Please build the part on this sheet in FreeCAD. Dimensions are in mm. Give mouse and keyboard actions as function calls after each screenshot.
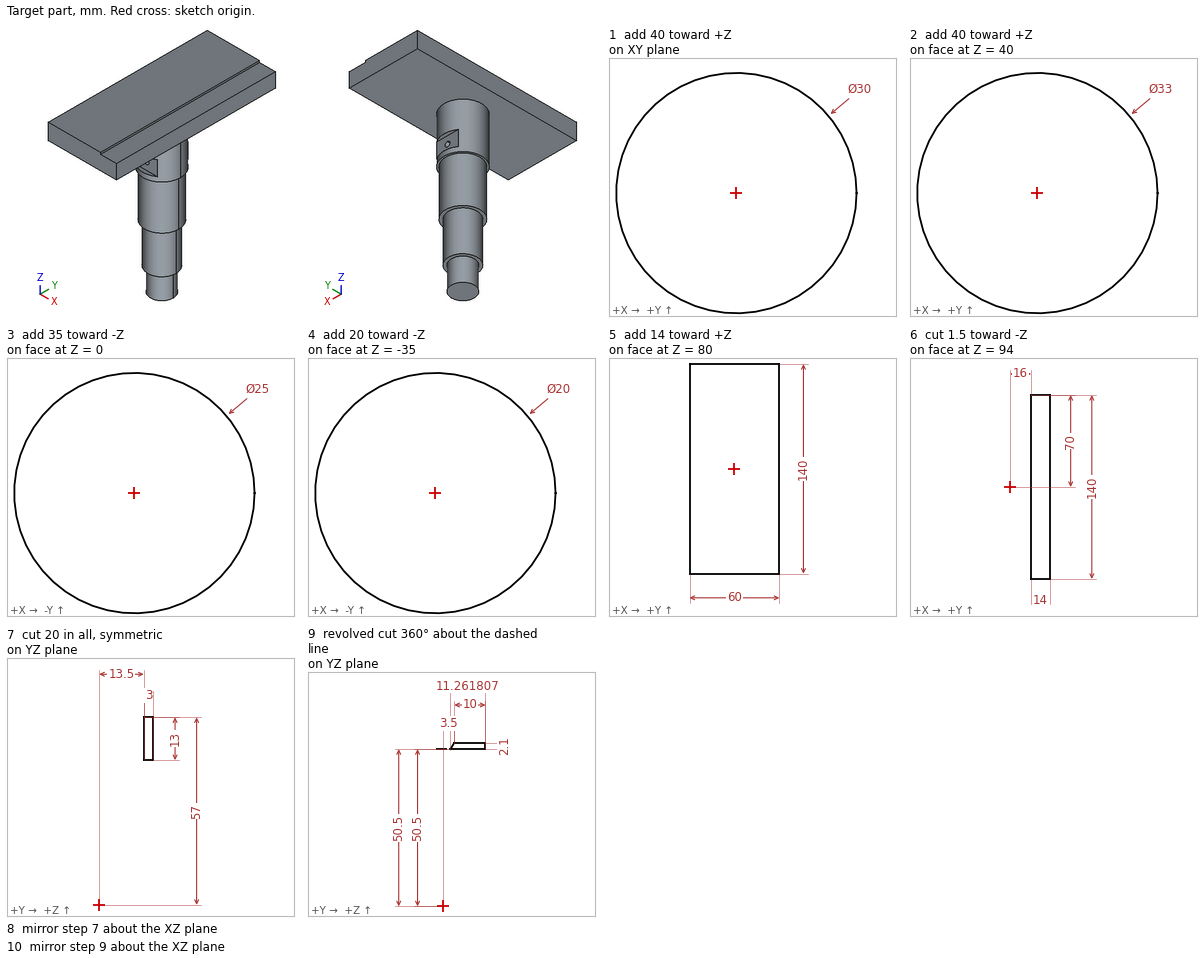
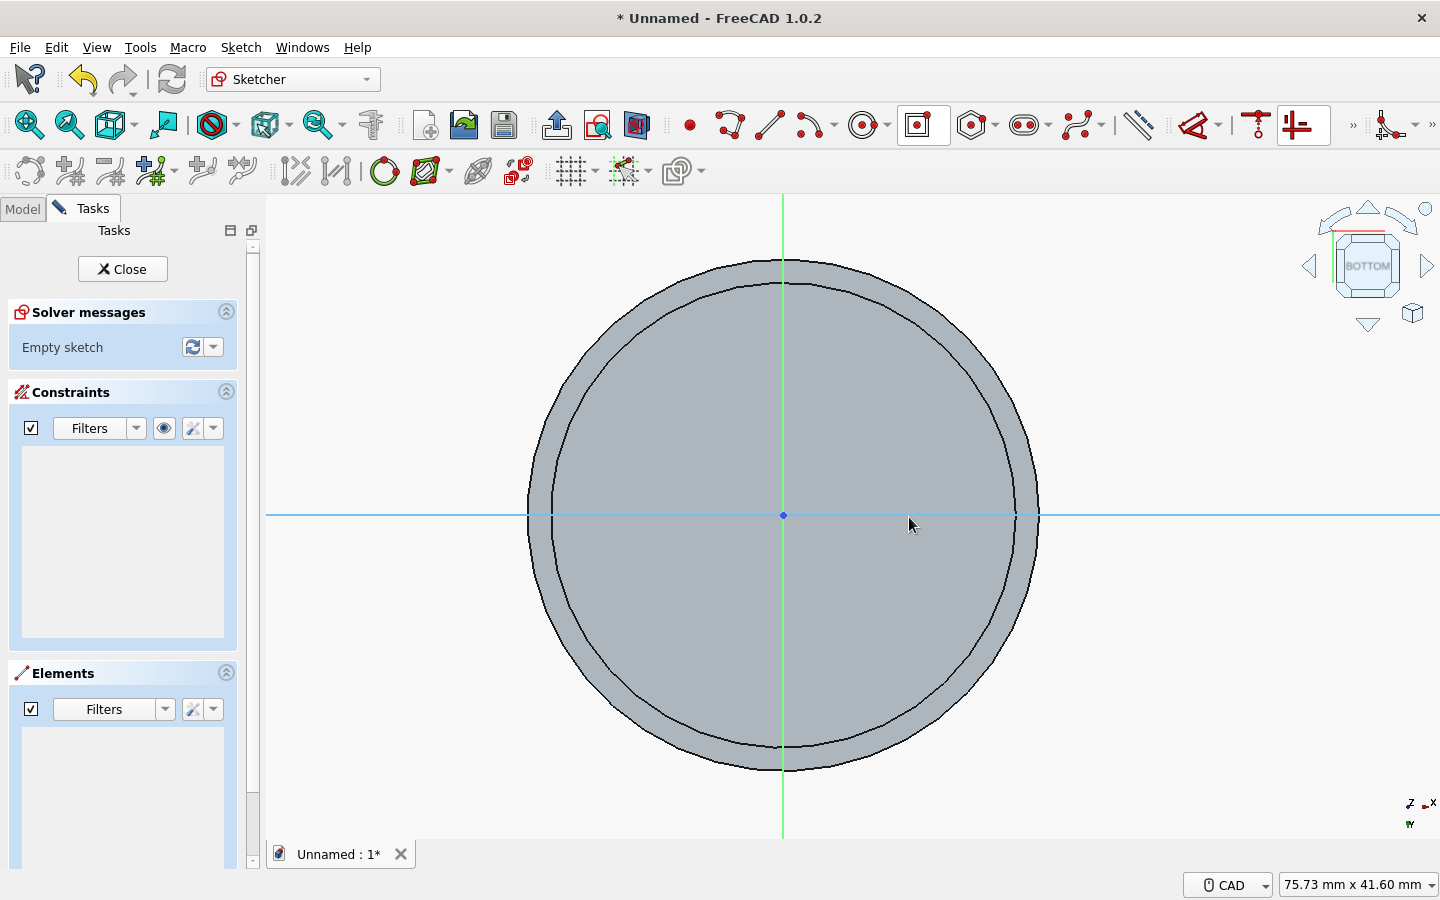
click(864, 126)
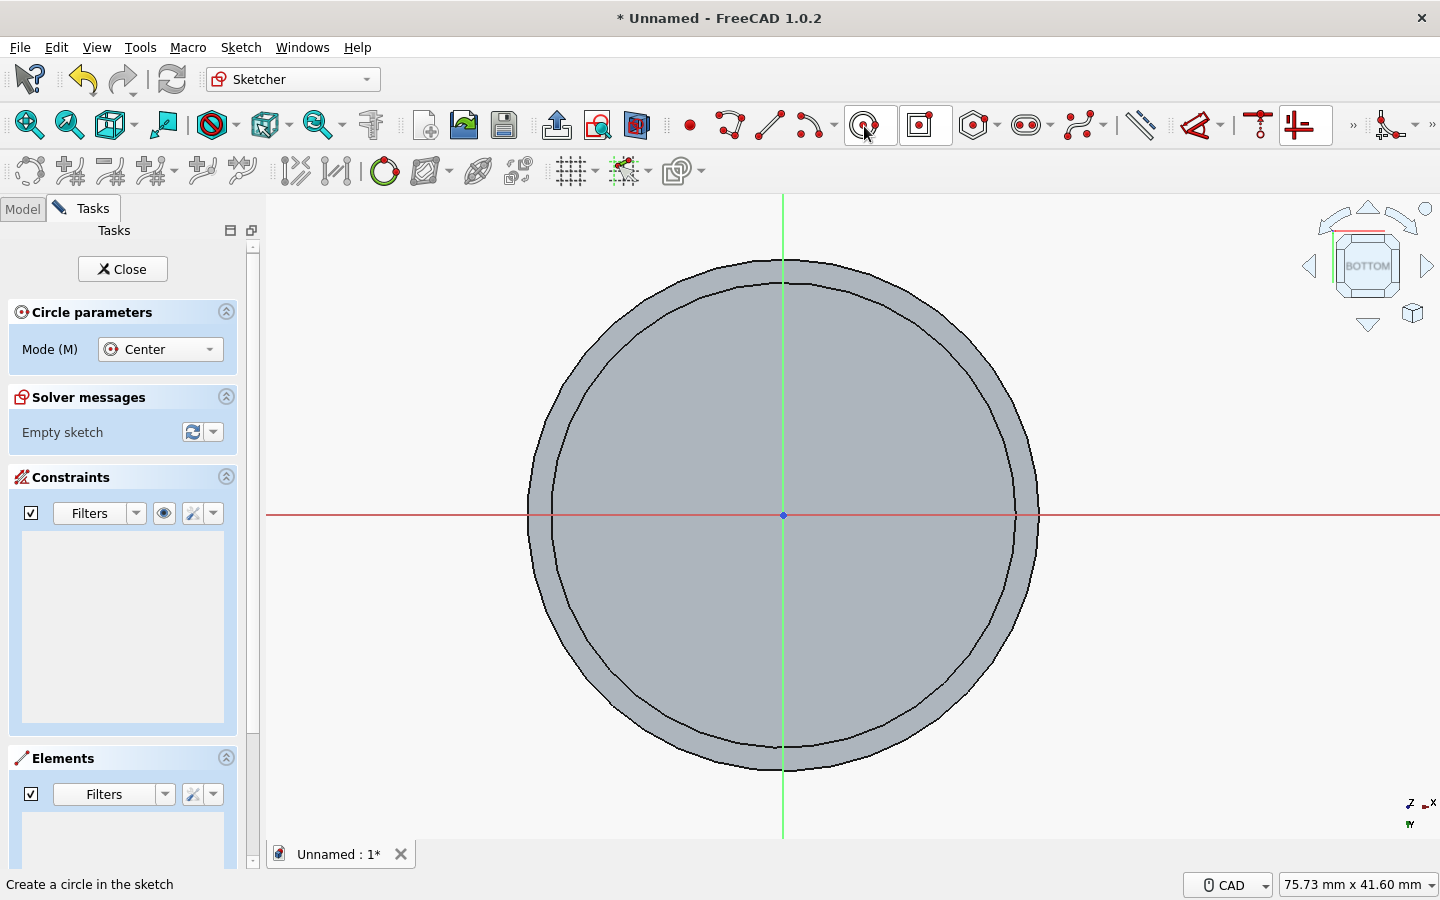
click(783, 515)
move(920, 378)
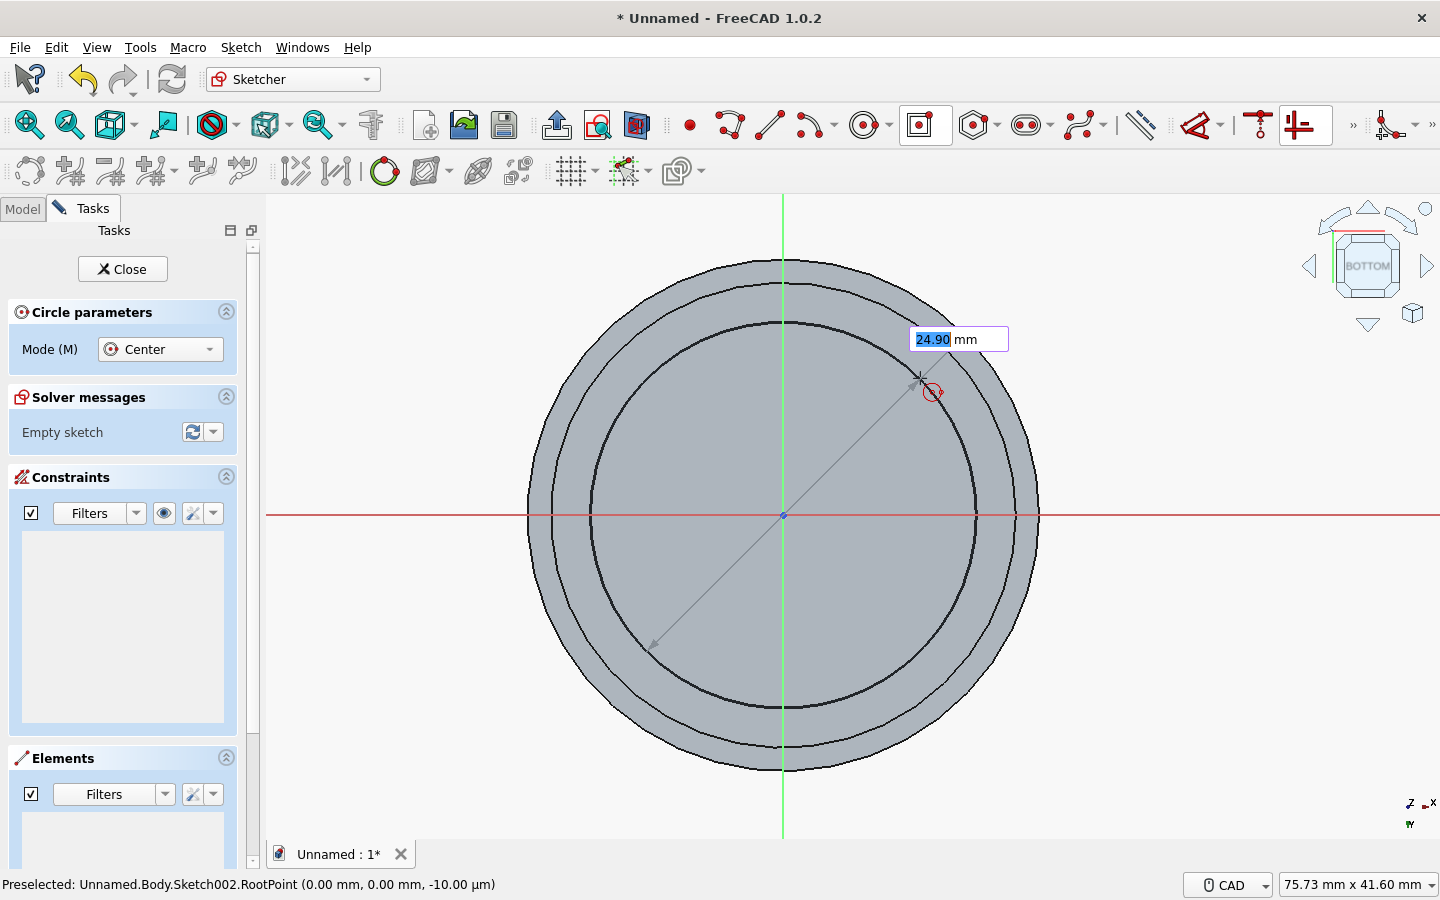
text(25)
key(Return)
key(Escape)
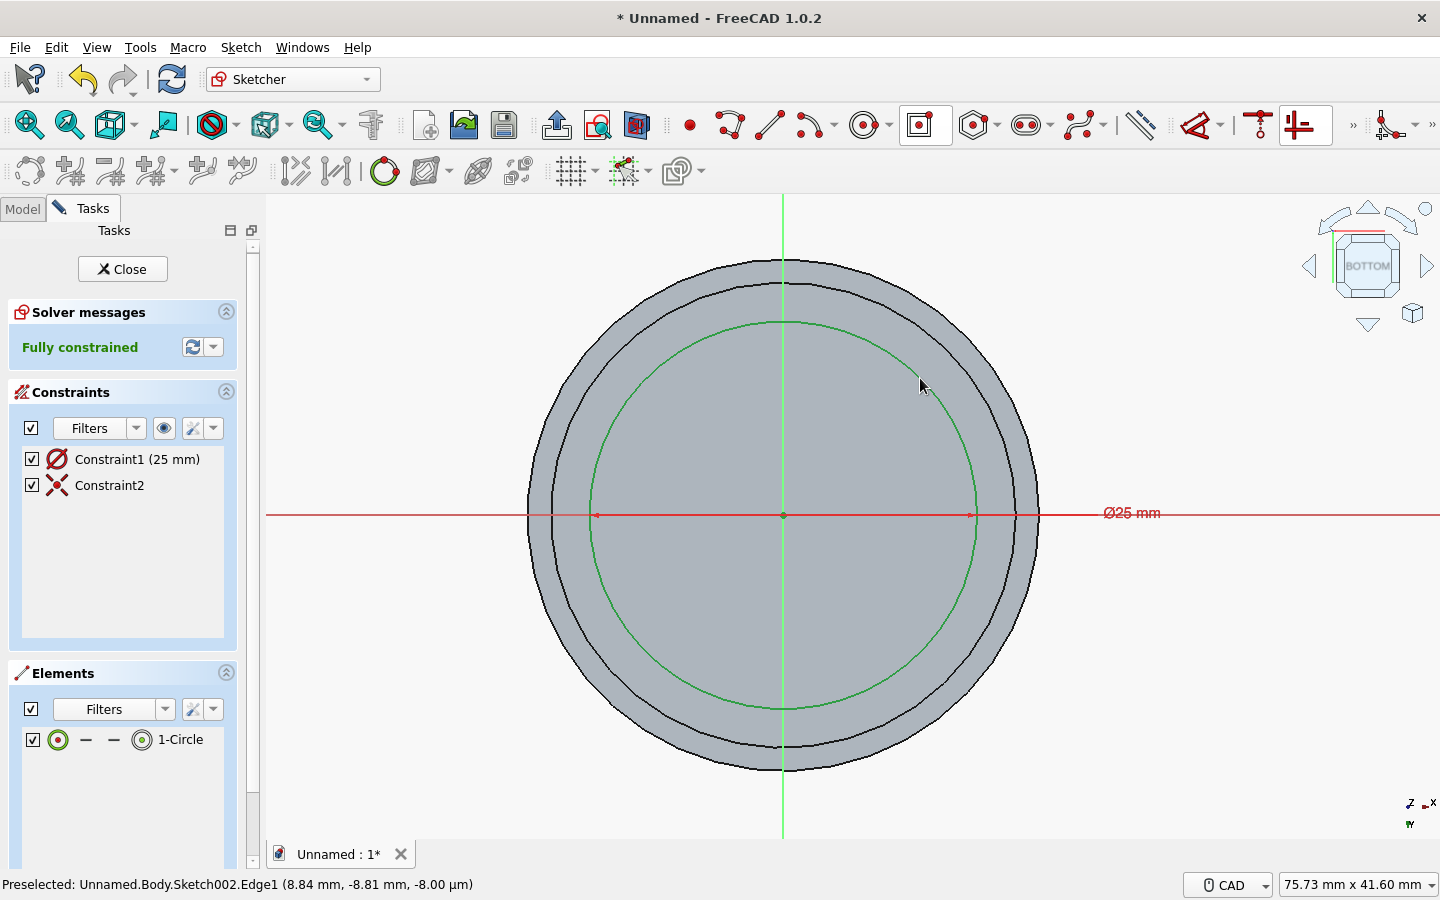
click(123, 269)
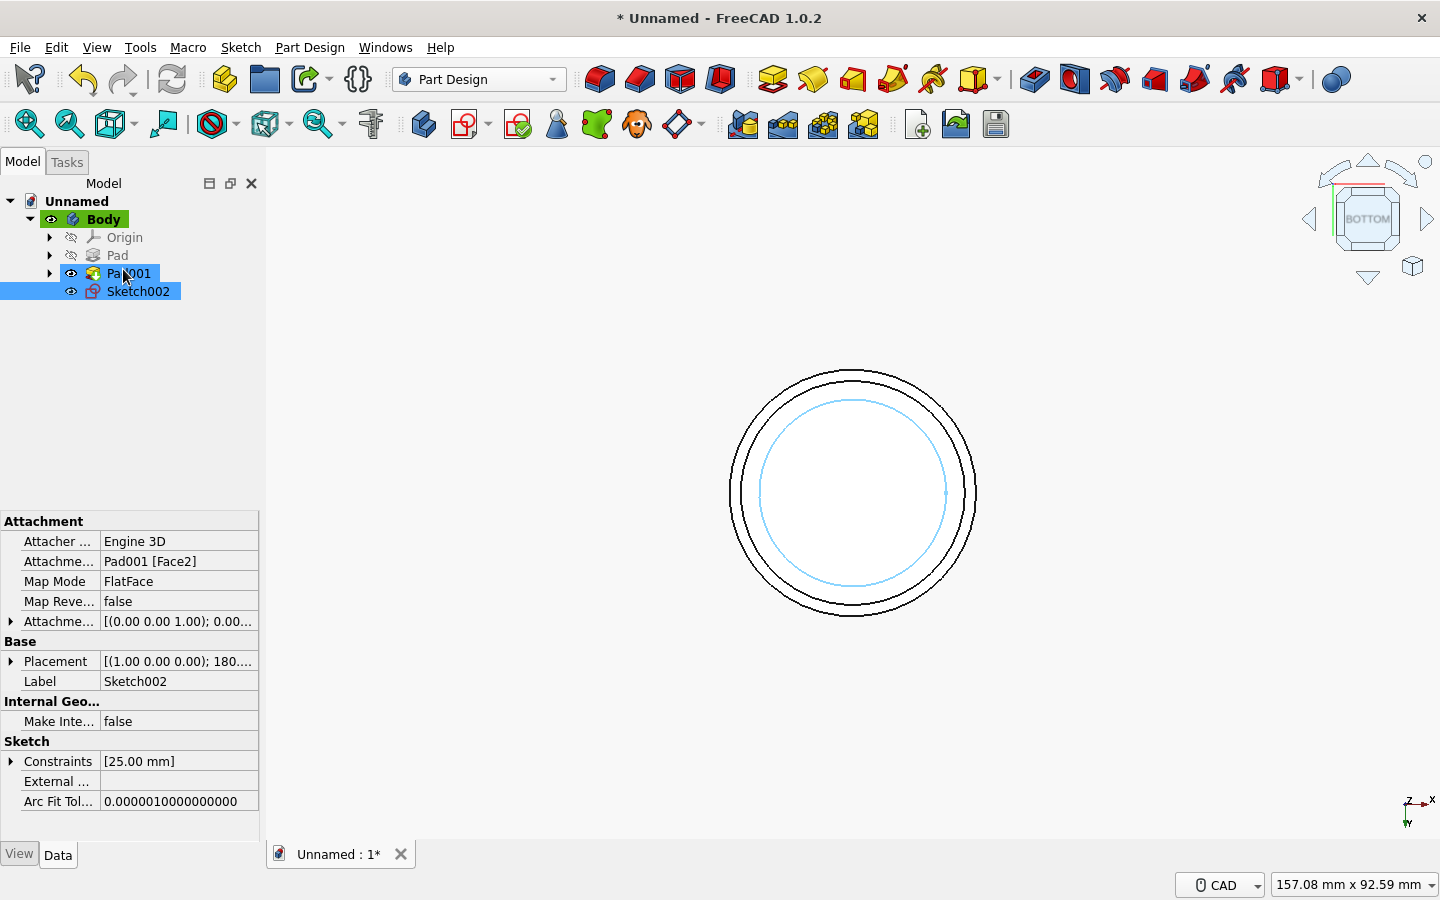
click(774, 80)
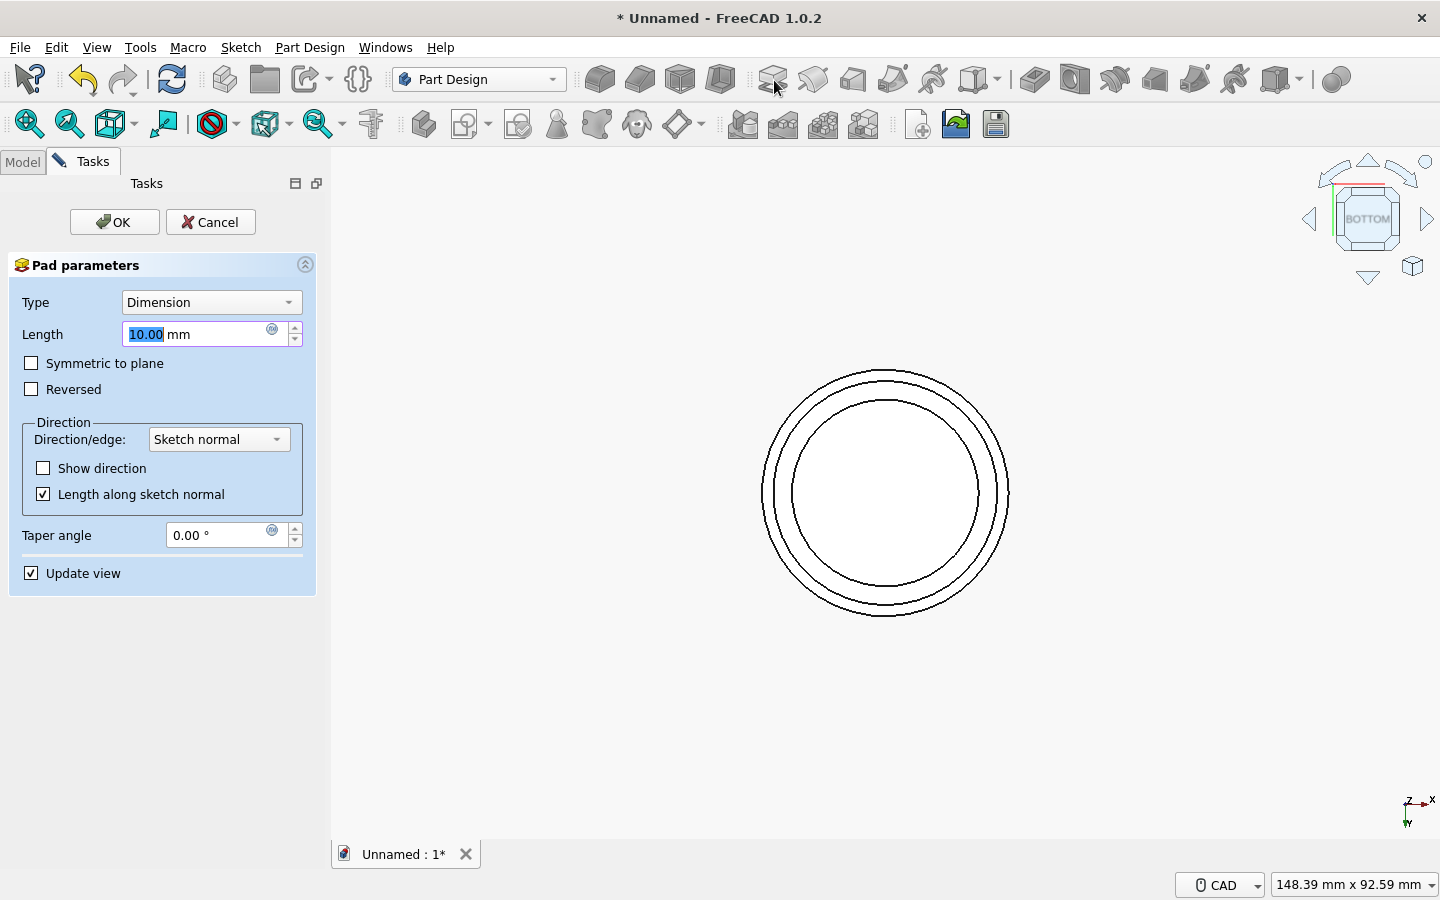
text(35)
key(Tab)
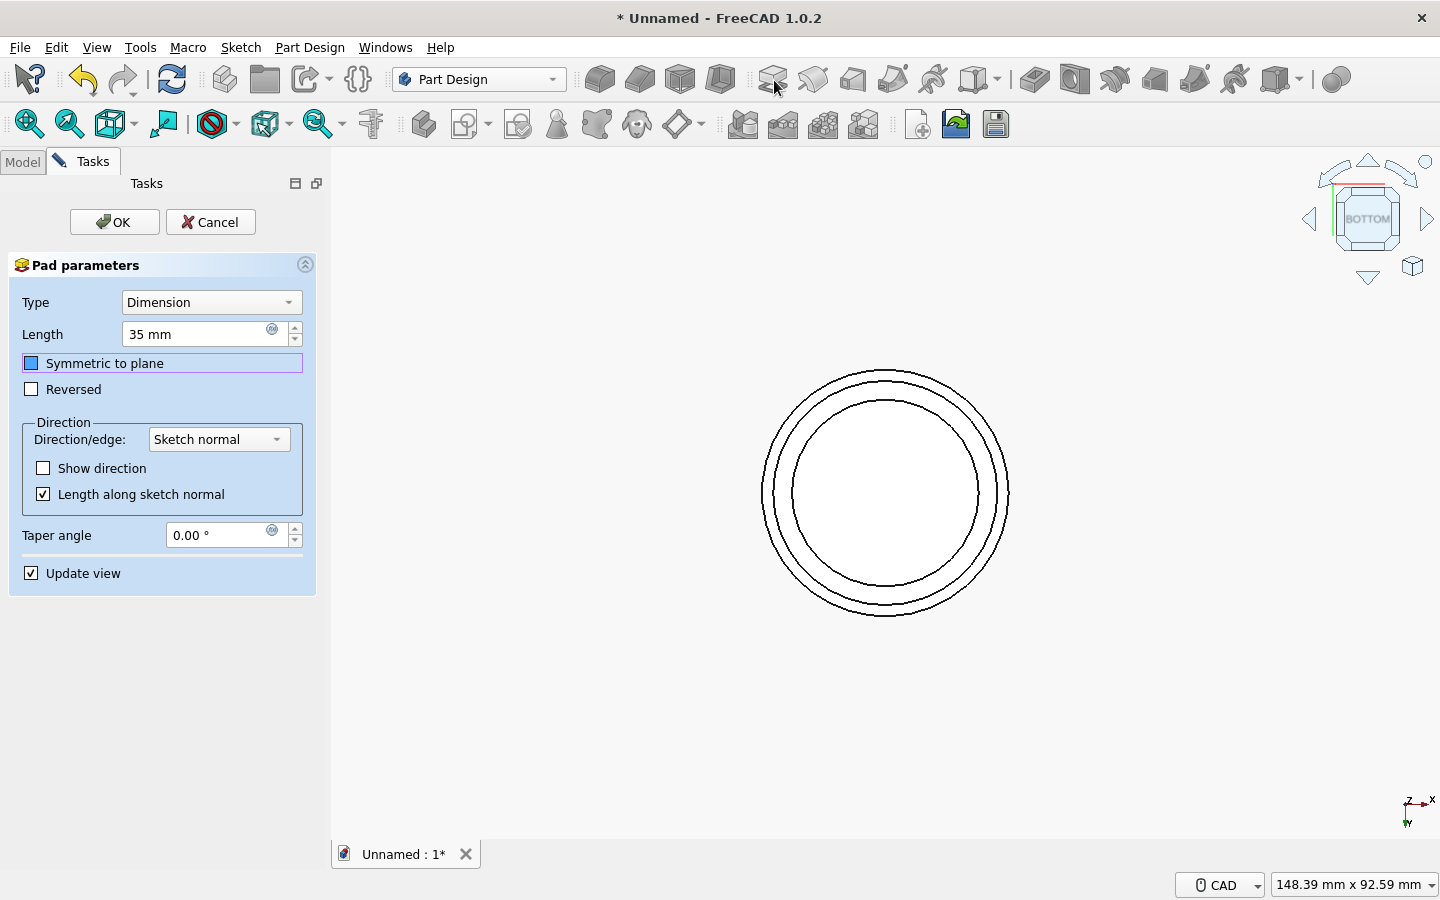
click(115, 222)